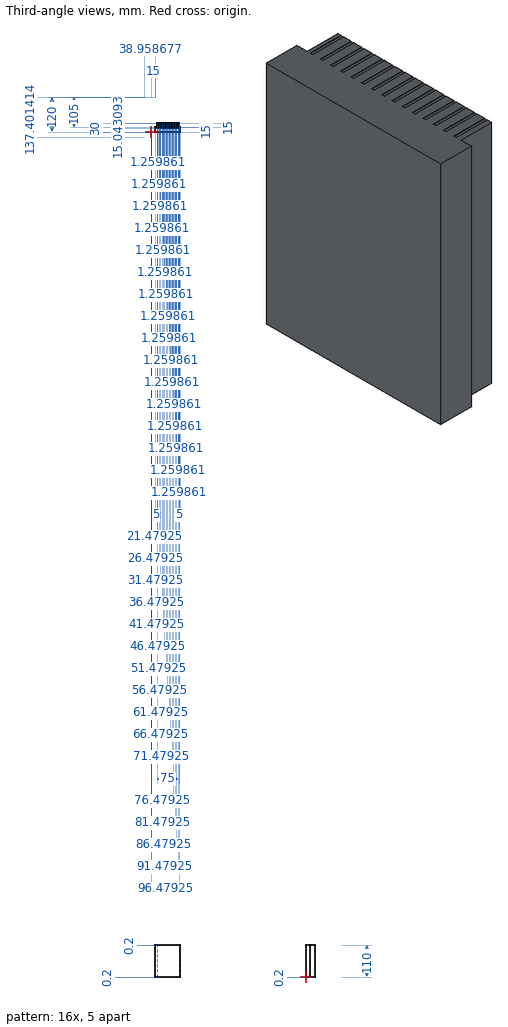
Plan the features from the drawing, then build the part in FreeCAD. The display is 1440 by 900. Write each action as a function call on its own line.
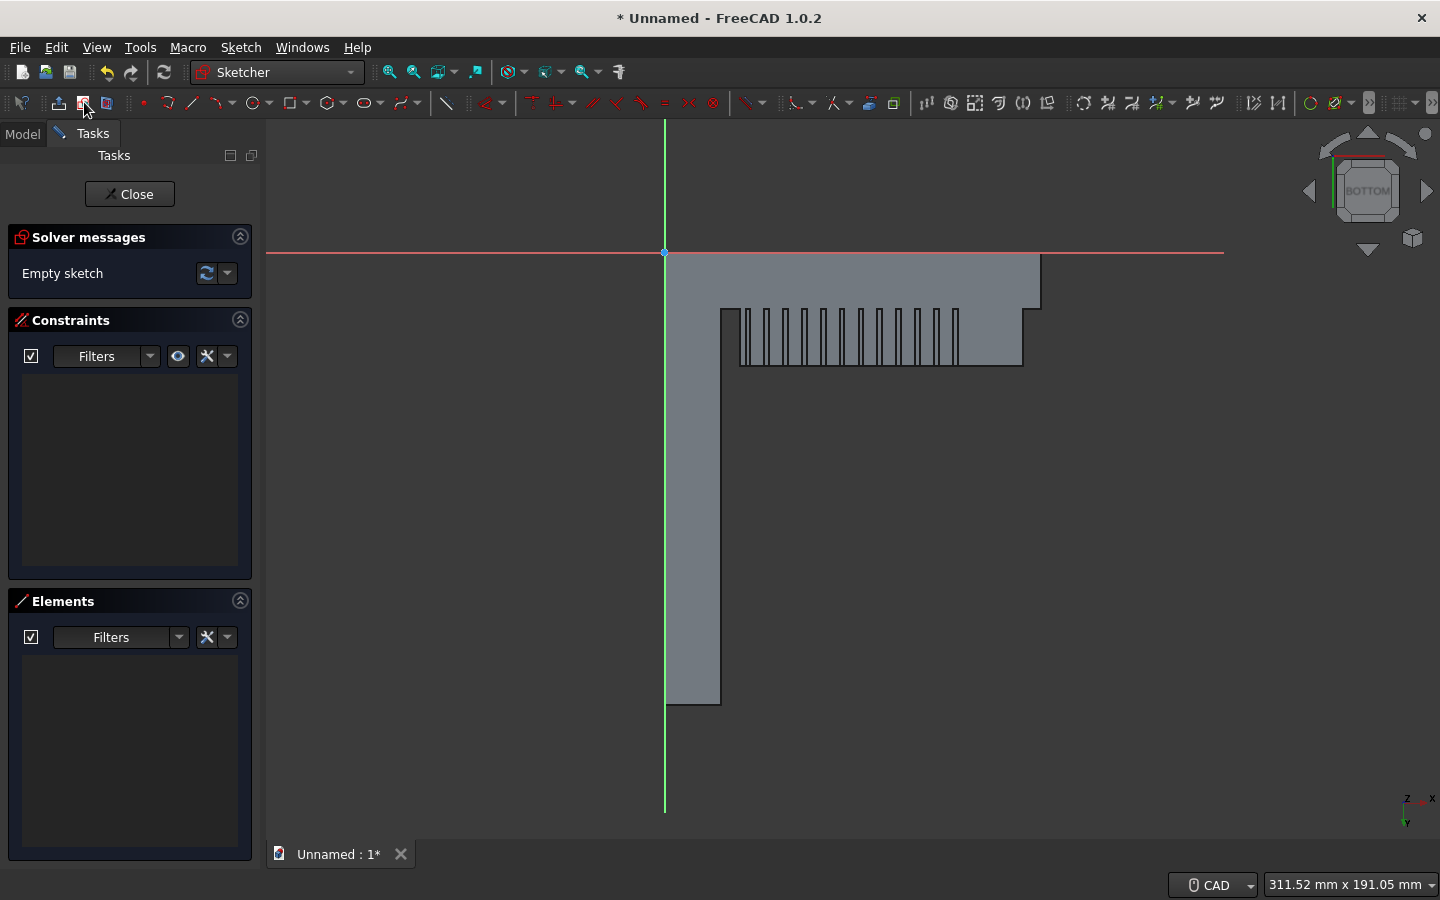
scroll(998, 320, up, 11)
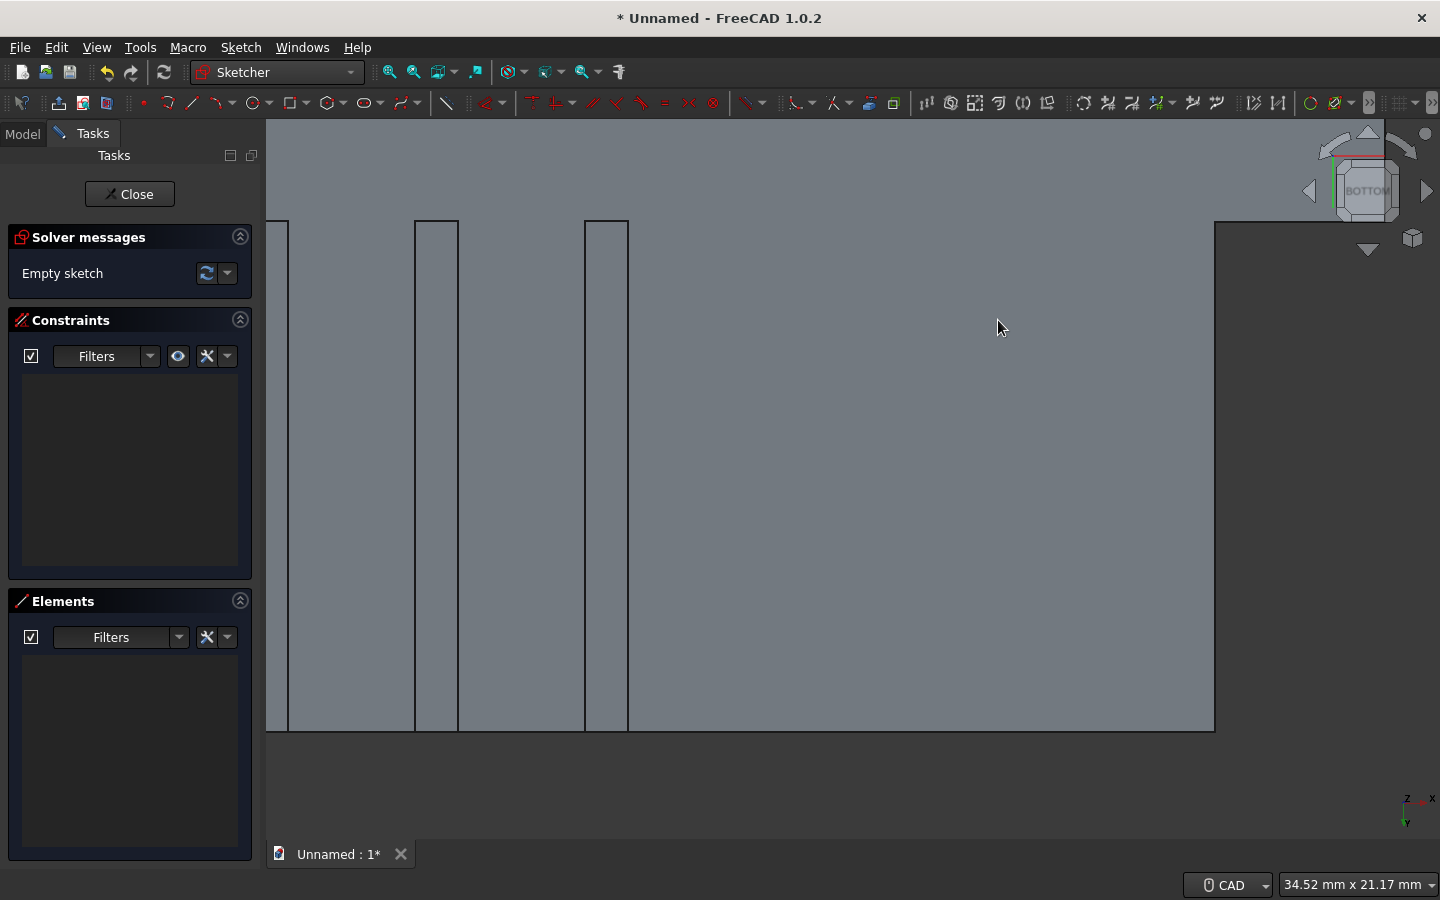
click(290, 104)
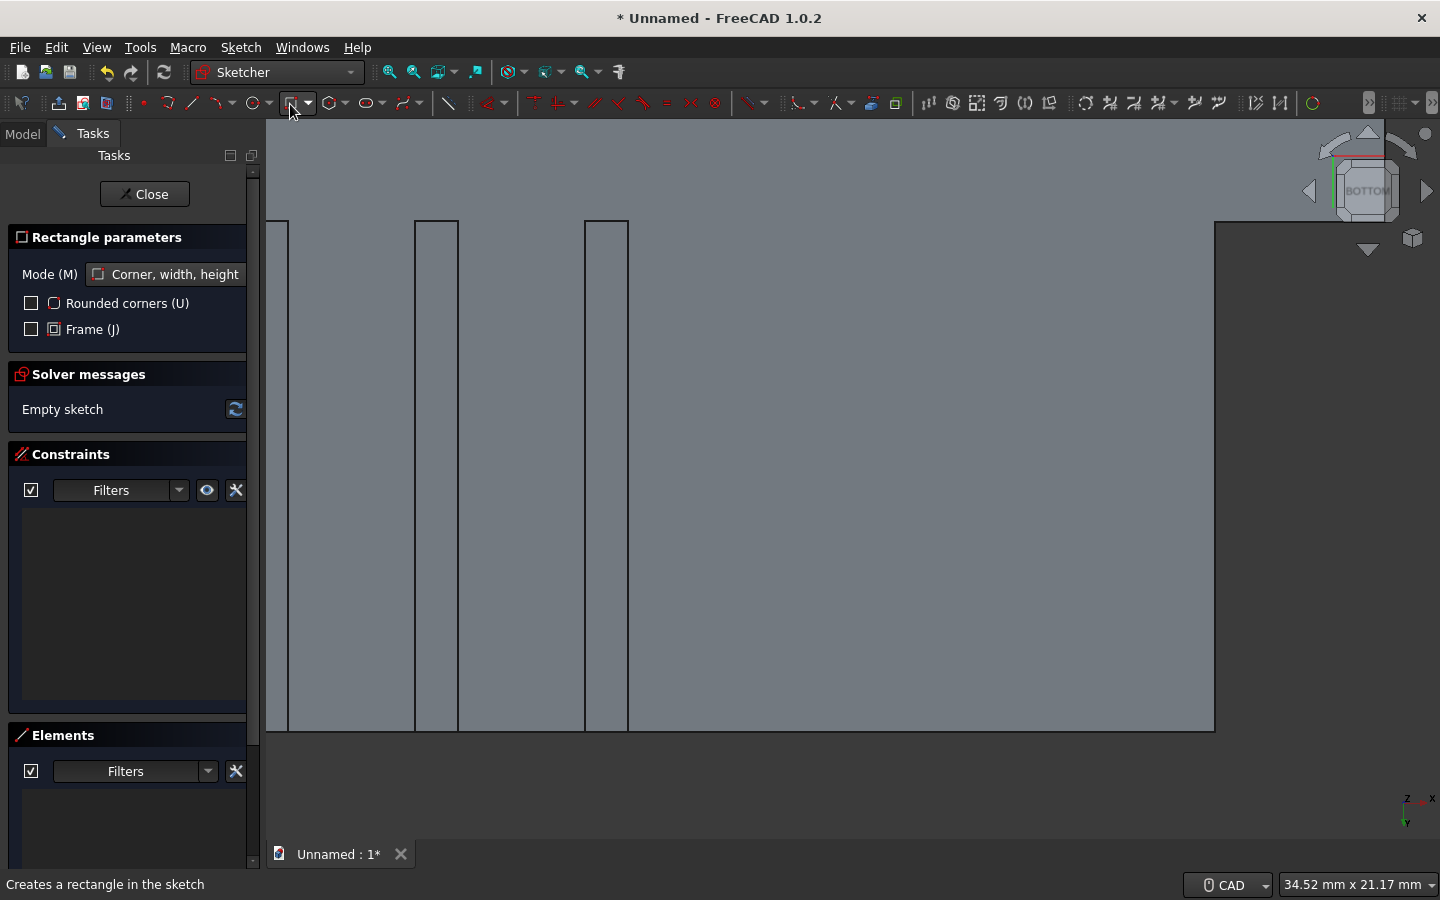
click(755, 221)
click(798, 732)
key(Escape)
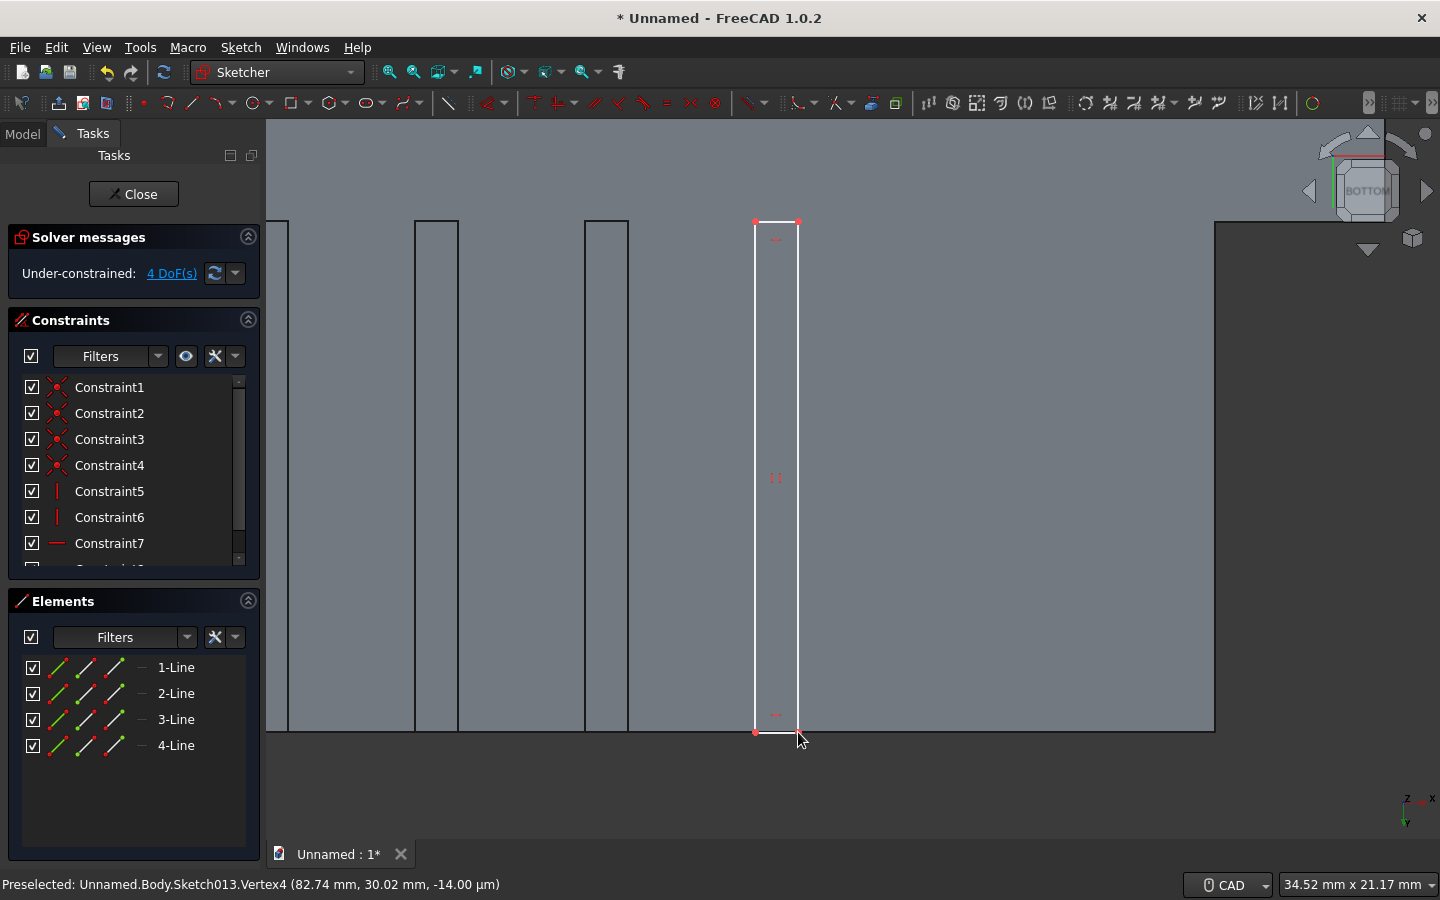
click(488, 104)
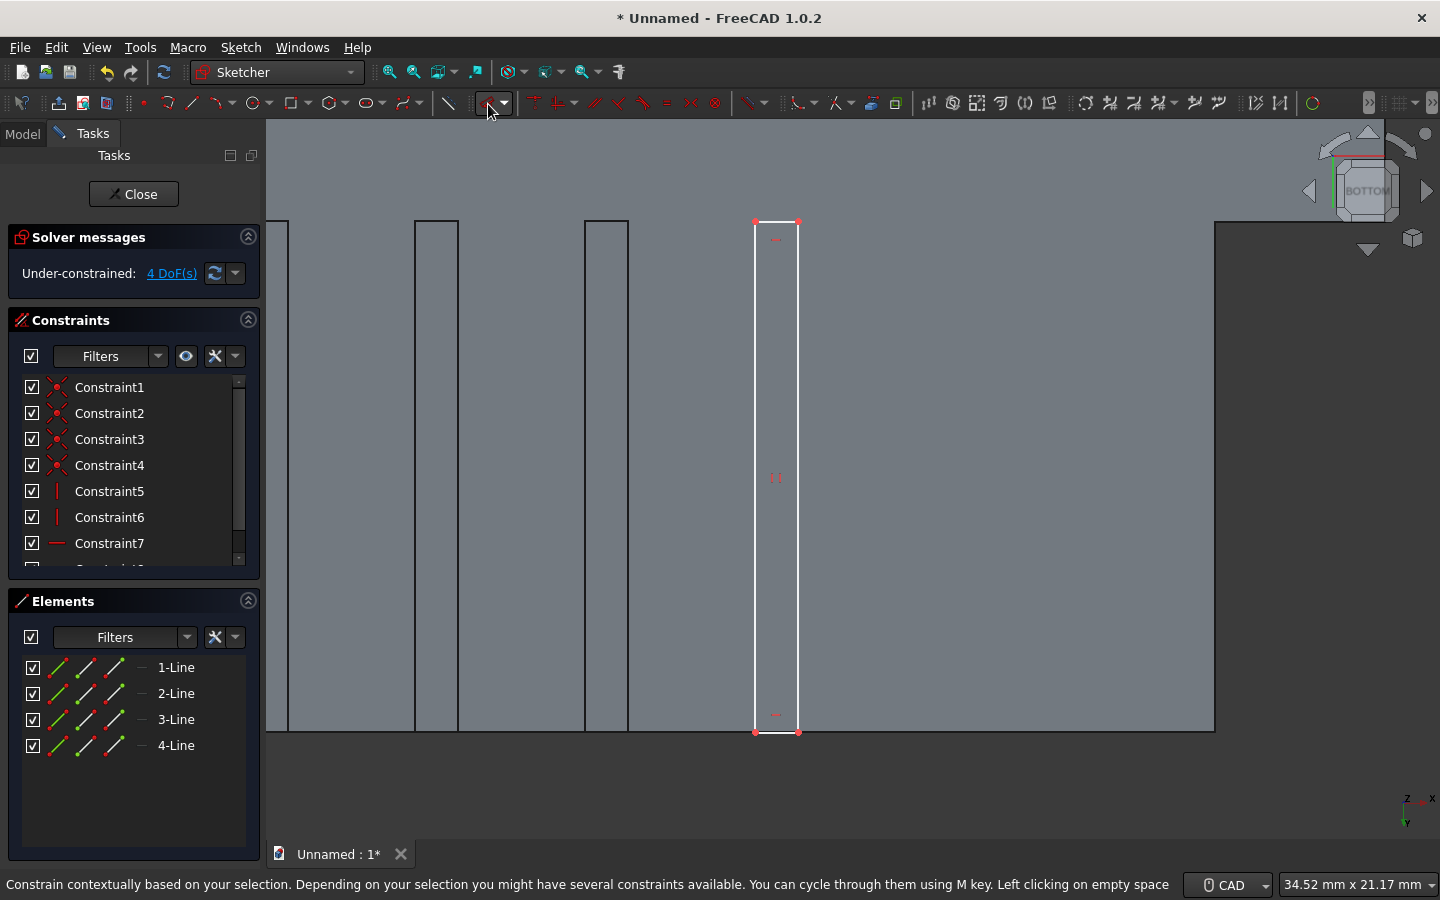
click(755, 733)
click(813, 440)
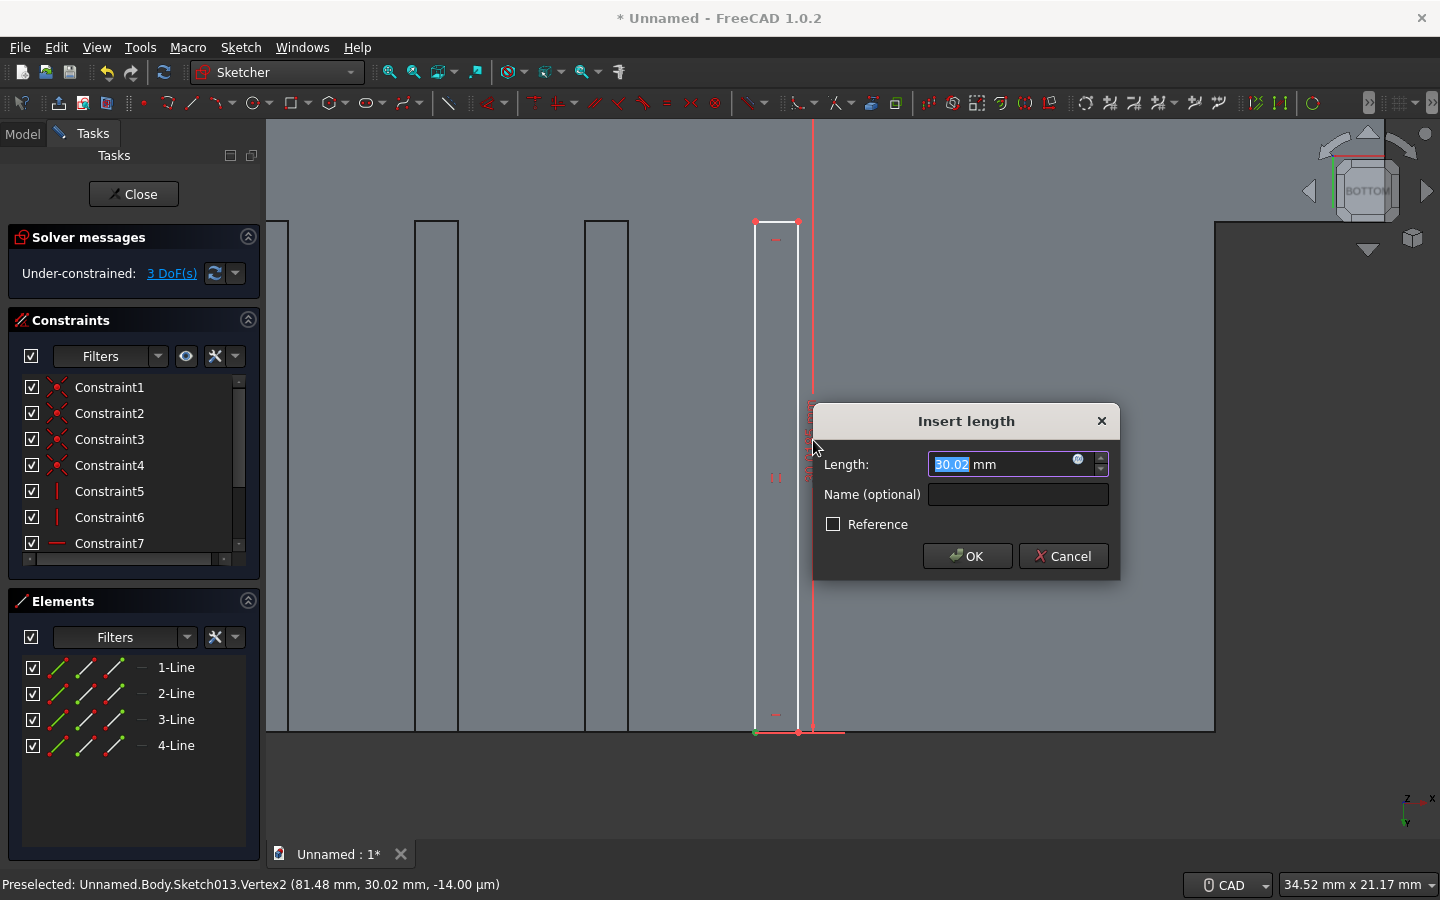
text(30)
key(Return)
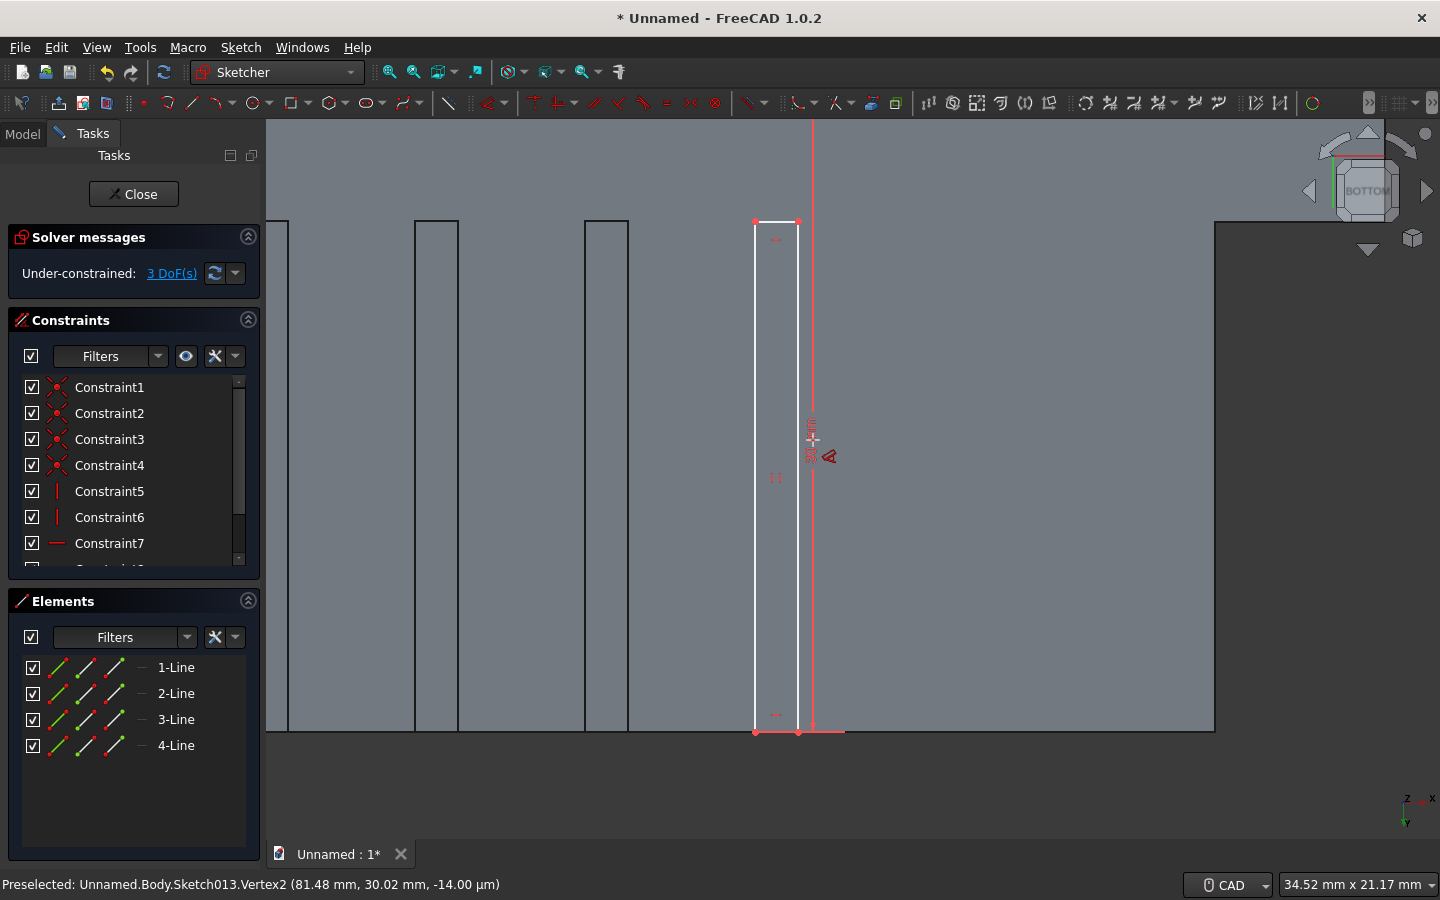
click(768, 732)
click(776, 766)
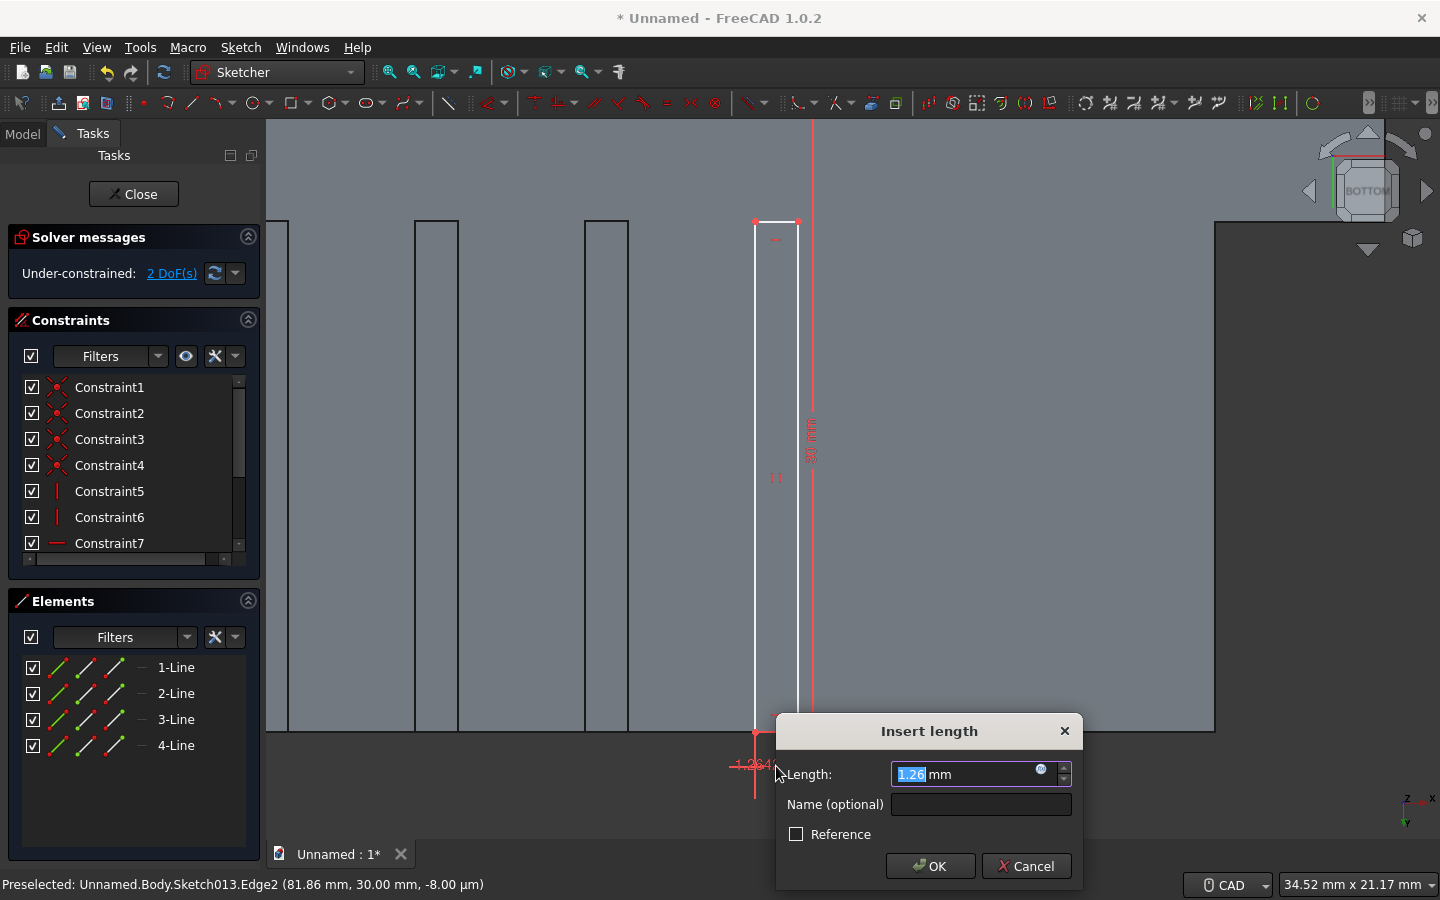
text(1.259861)
key(Return)